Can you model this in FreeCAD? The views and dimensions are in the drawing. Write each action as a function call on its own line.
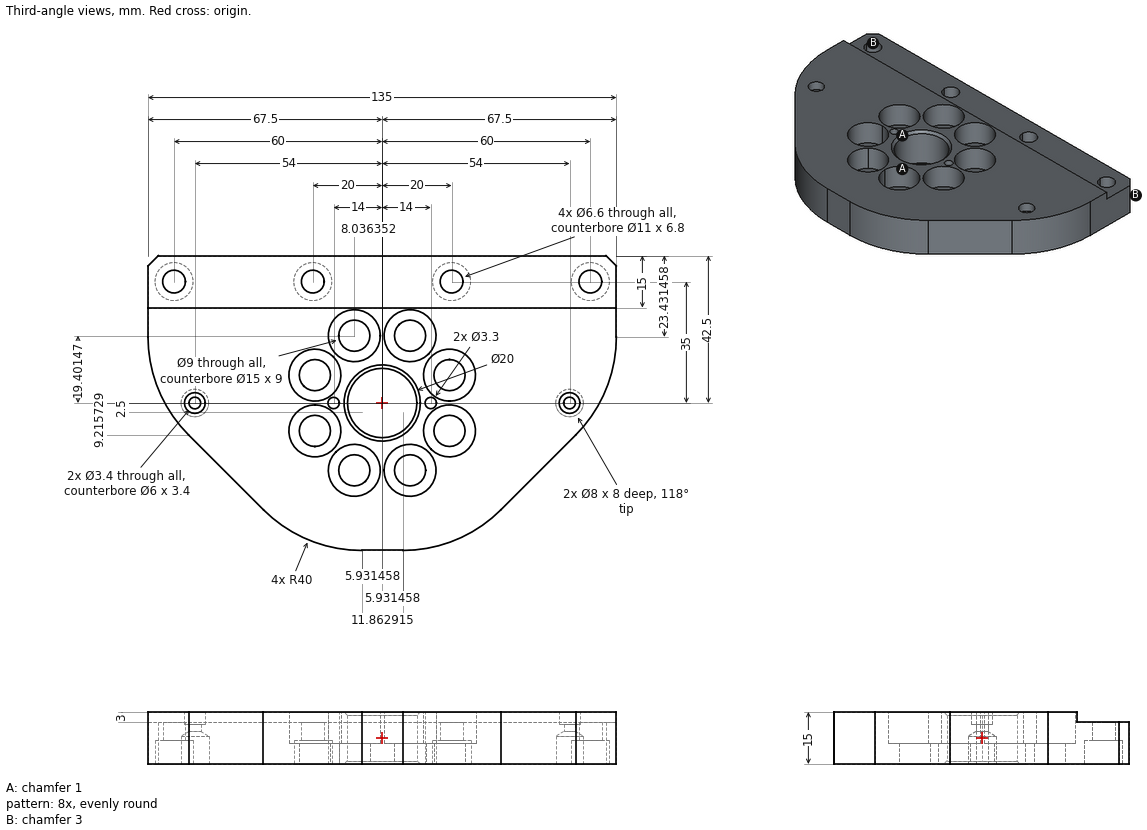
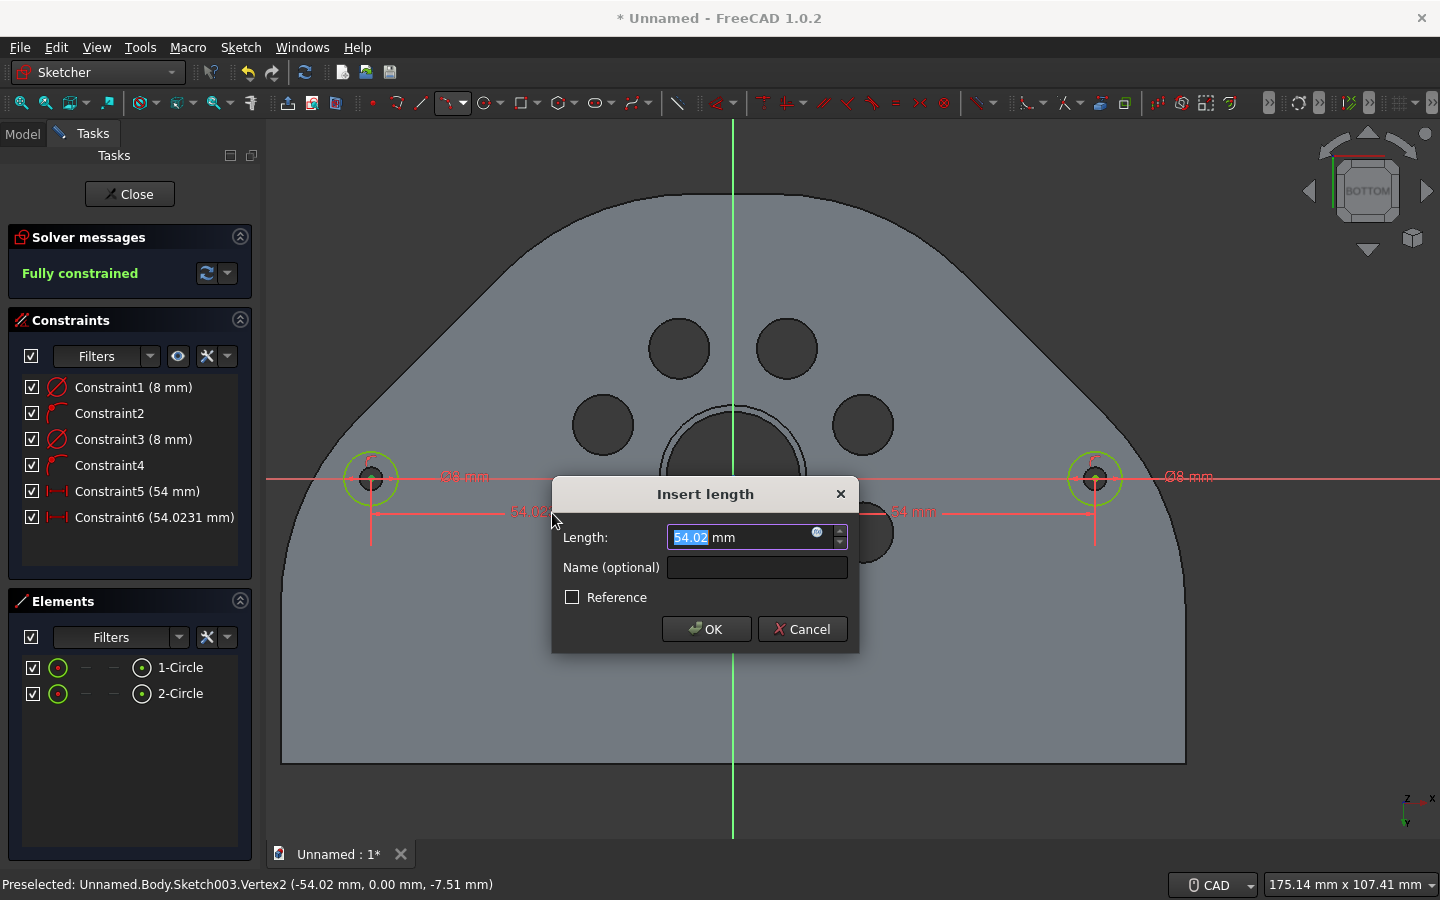
text(54)
key(Return)
key(Escape)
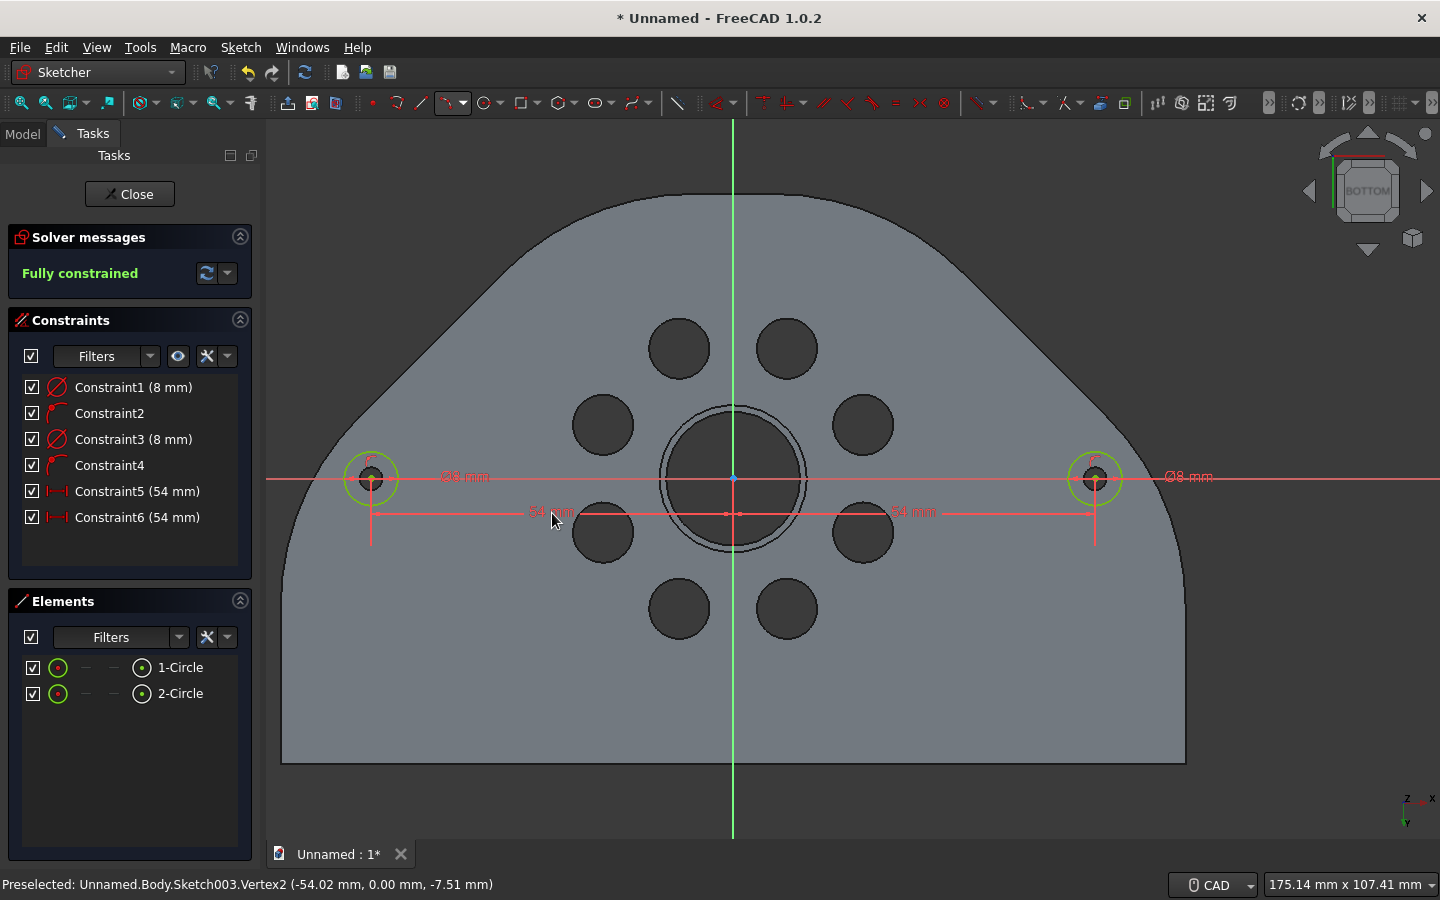
click(130, 194)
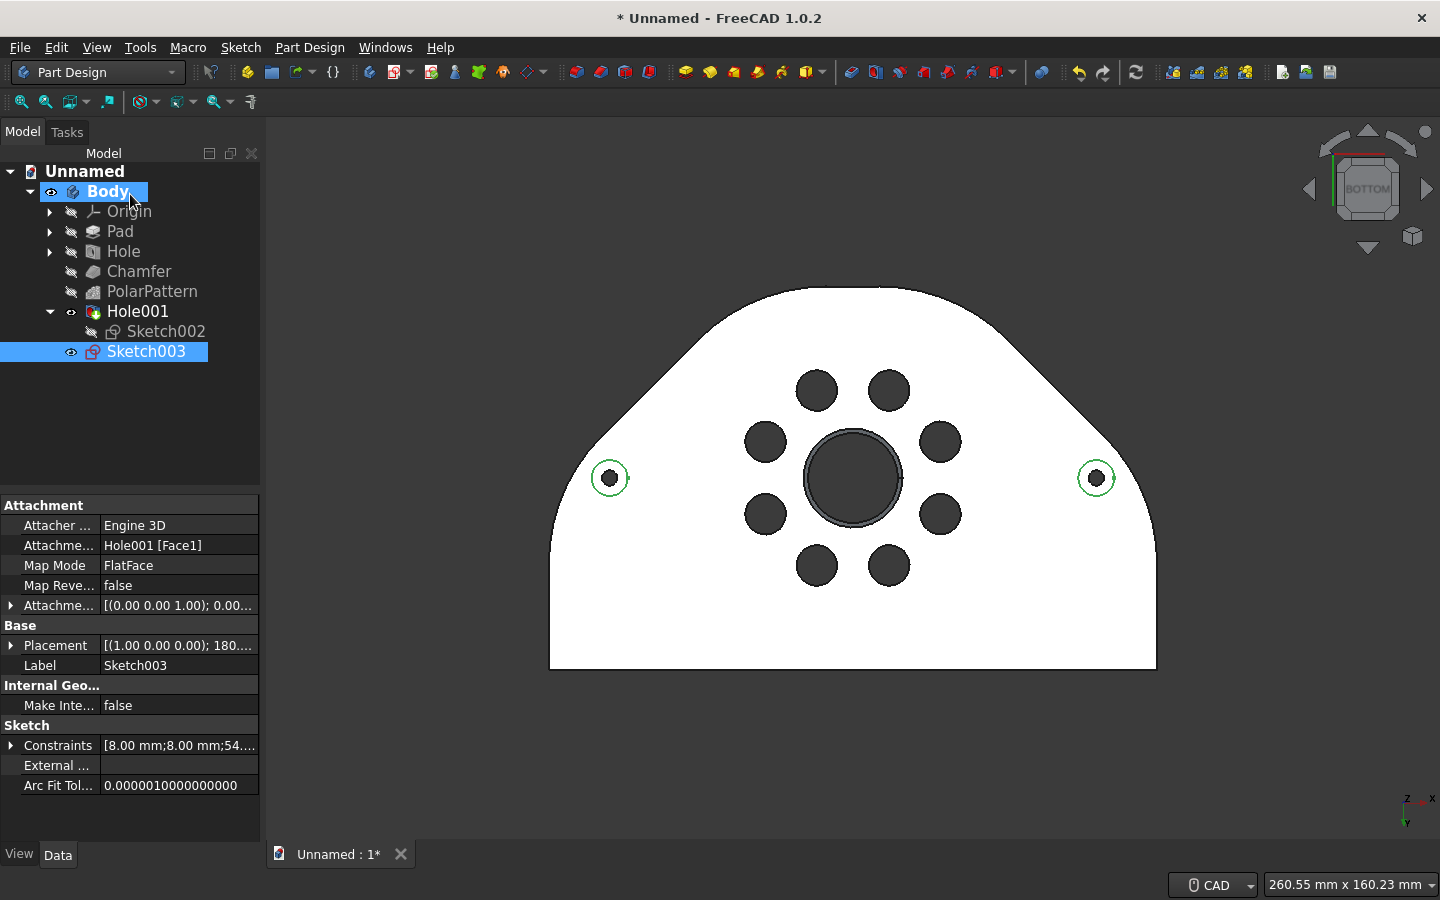
click(876, 72)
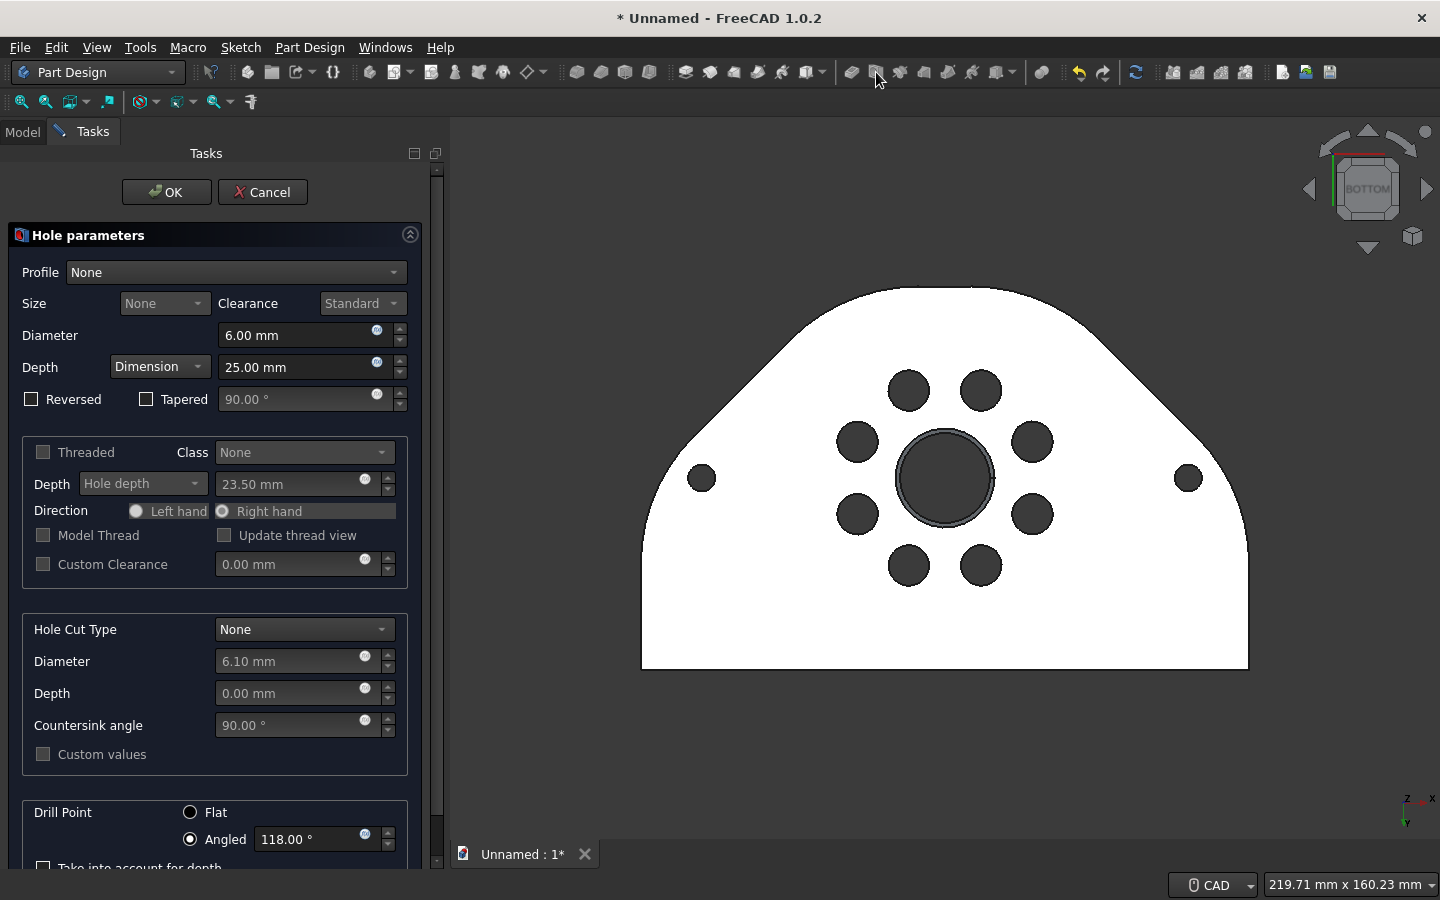
triple_click(305, 335)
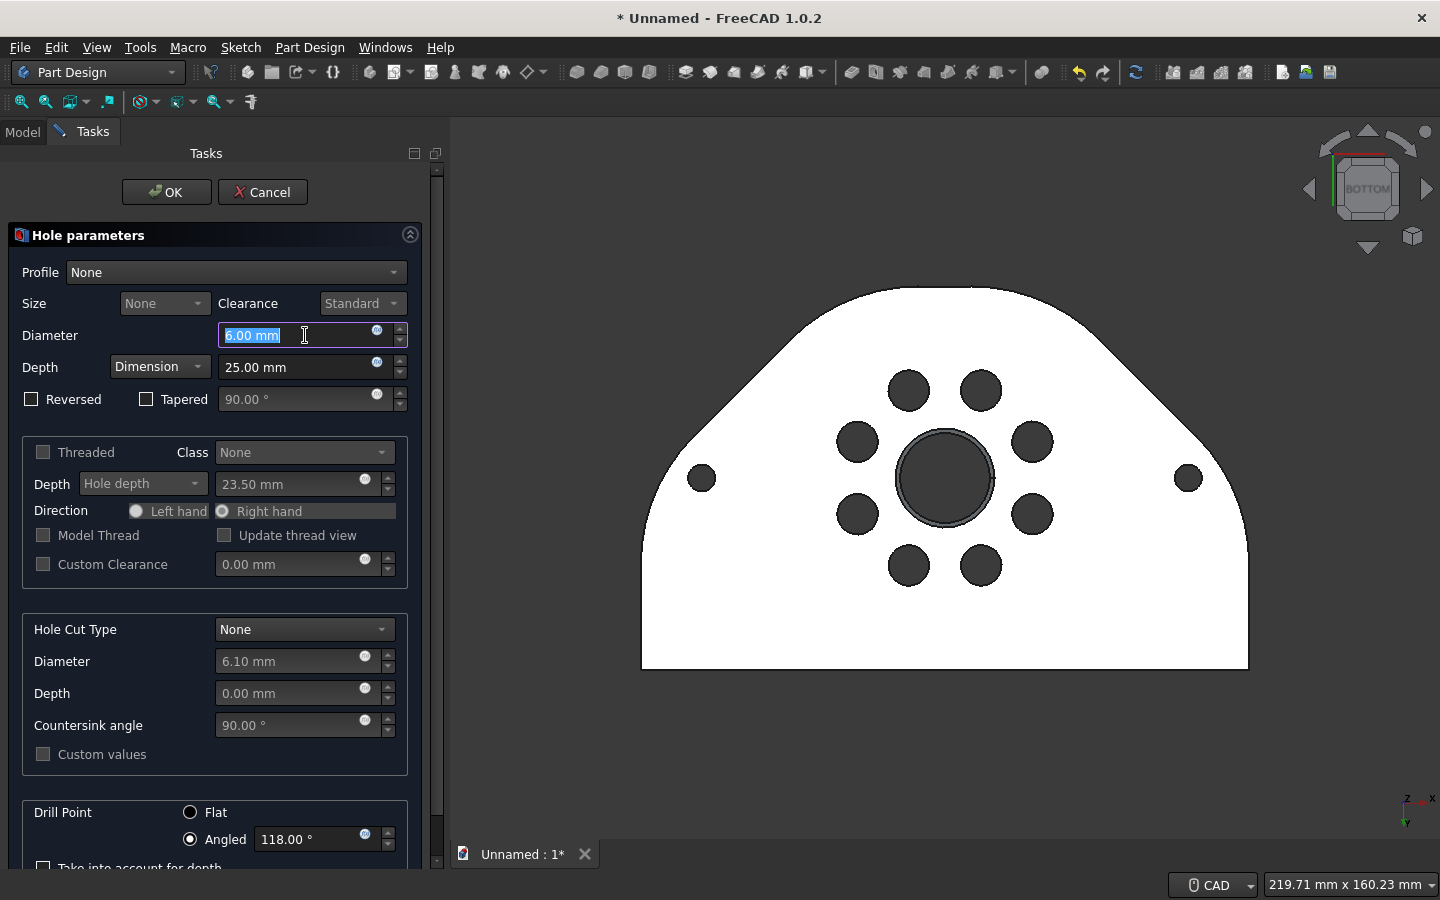
text(8)
key(Tab)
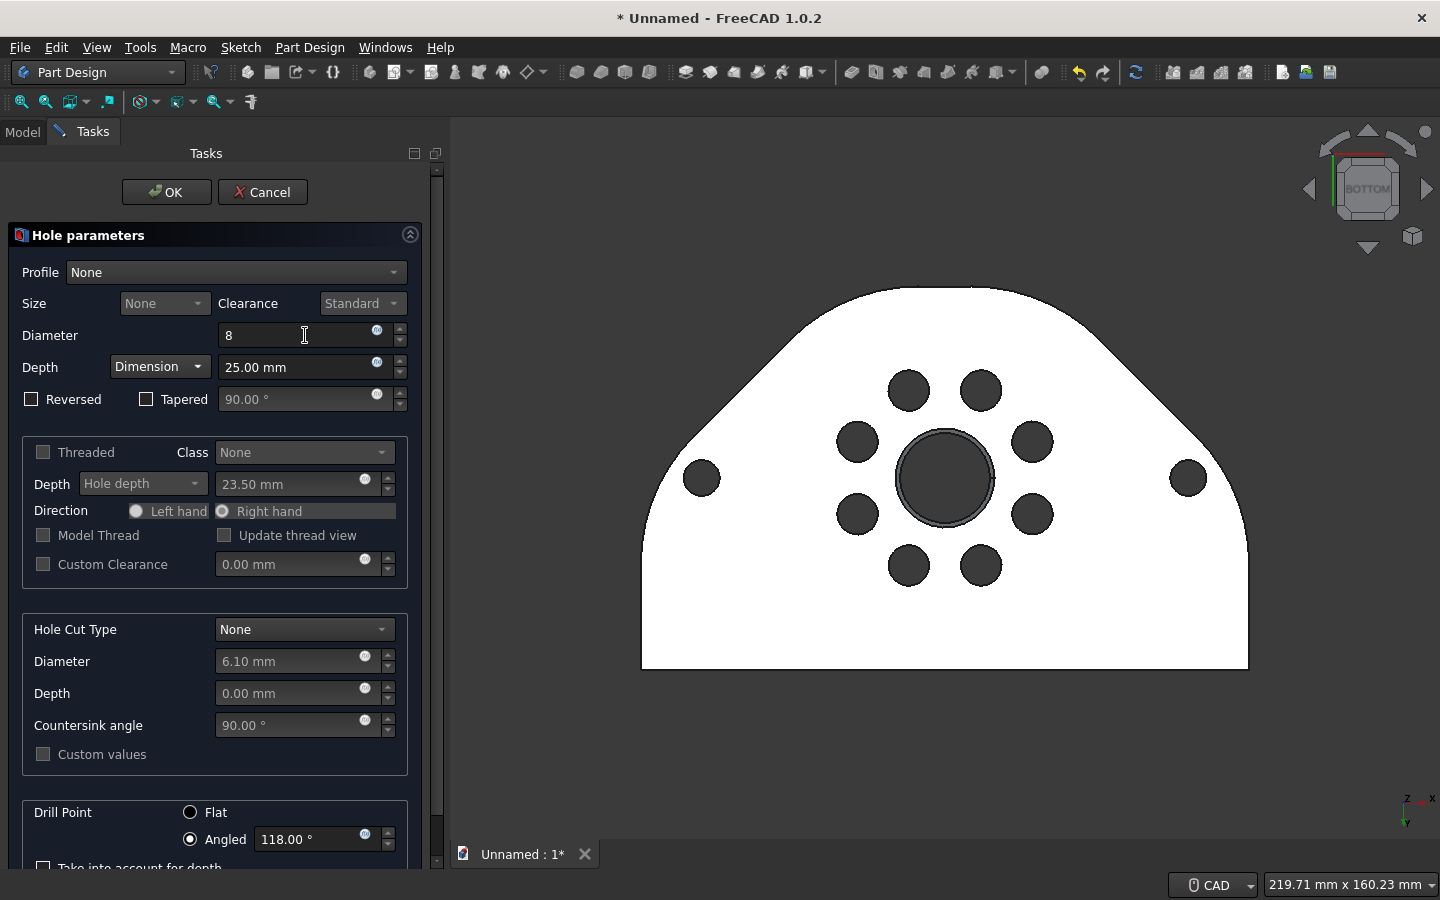
triple_click(305, 367)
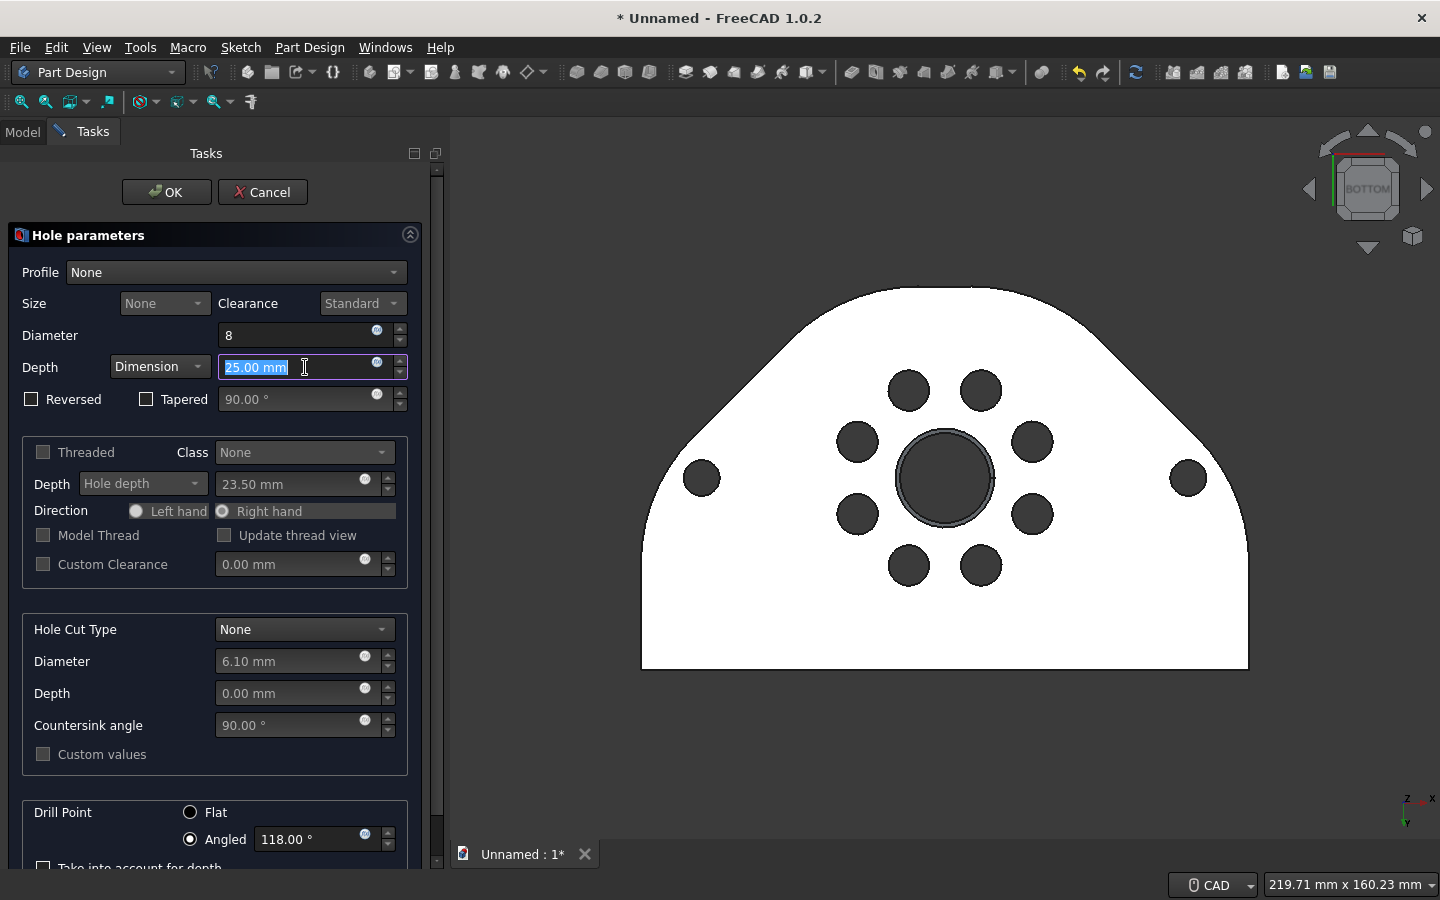
text(8)
key(Tab)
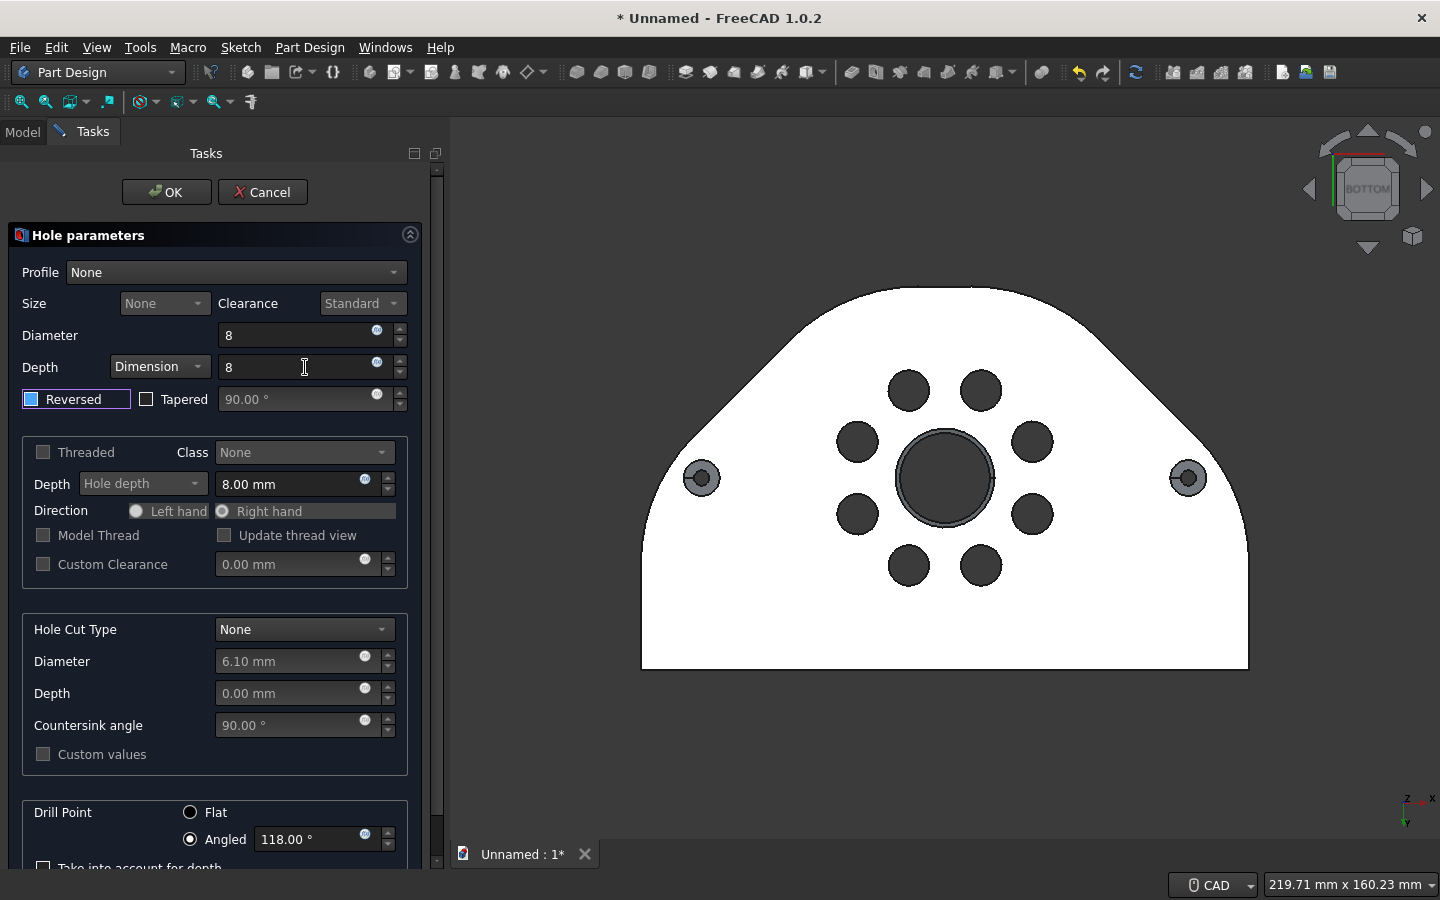
click(167, 192)